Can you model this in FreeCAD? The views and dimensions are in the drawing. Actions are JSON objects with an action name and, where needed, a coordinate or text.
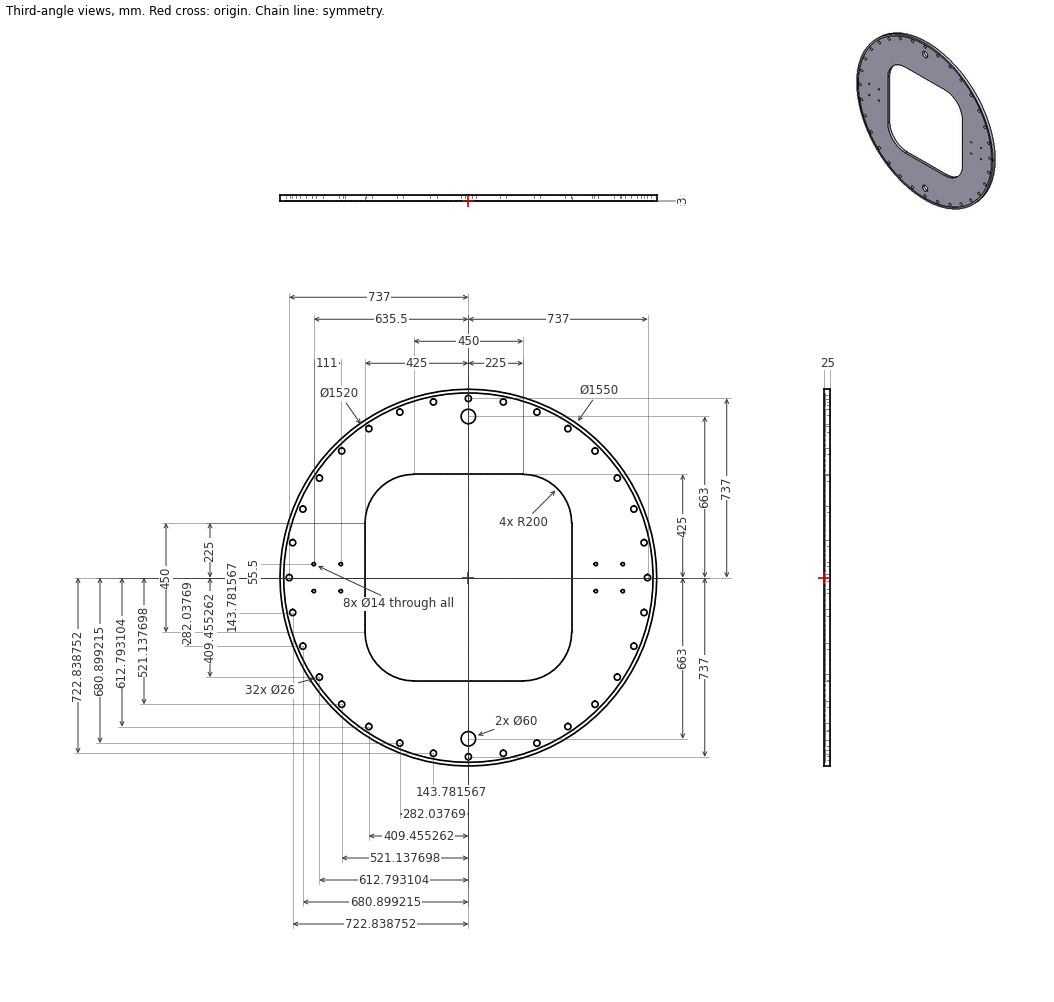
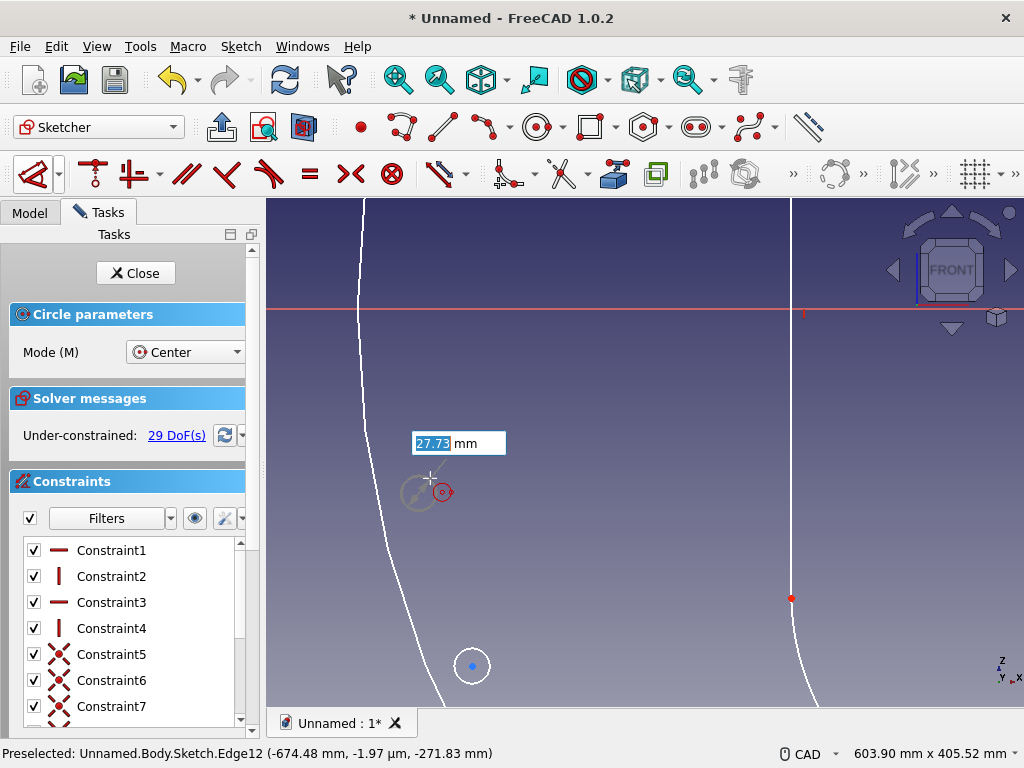
{"action": "left_click", "coordinate": [430, 478]}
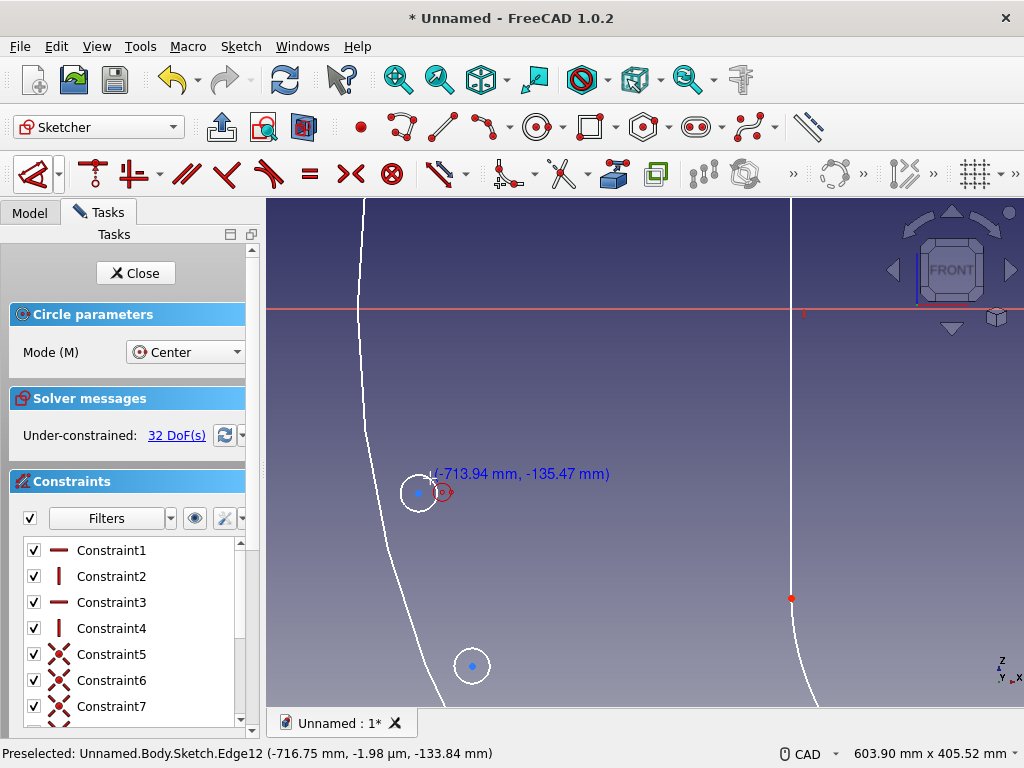
{"action": "scroll", "coordinate": [428, 481], "scroll_direction": "down", "scroll_amount": 9}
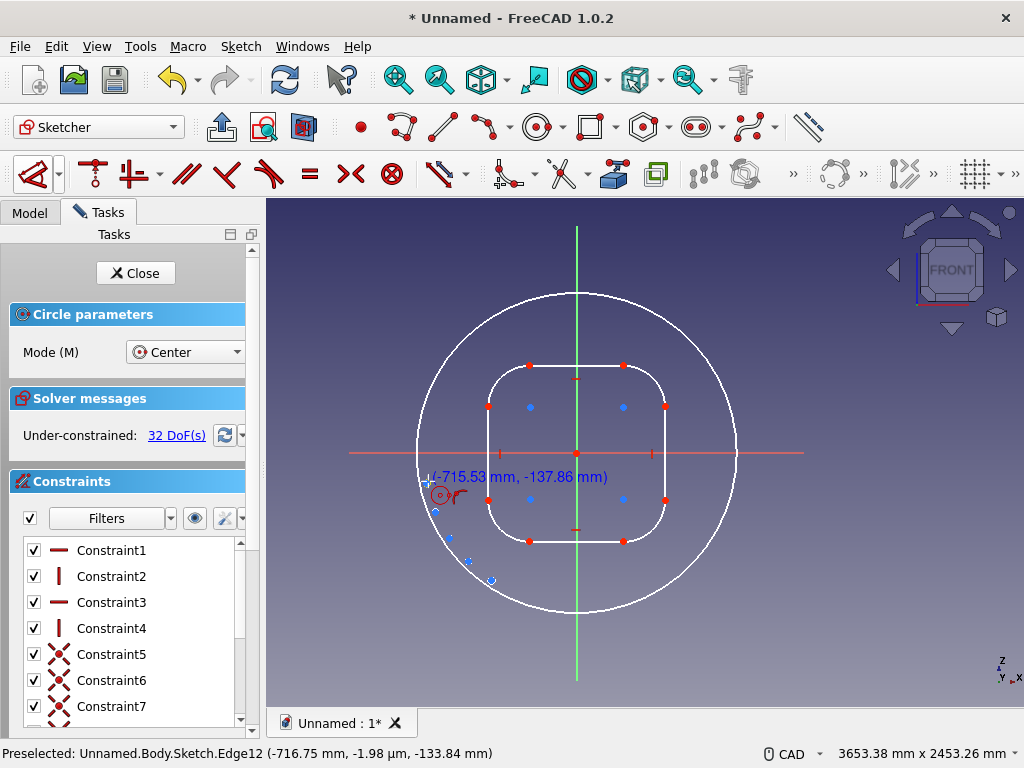
{"action": "scroll", "coordinate": [518, 594], "scroll_direction": "up", "scroll_amount": 11}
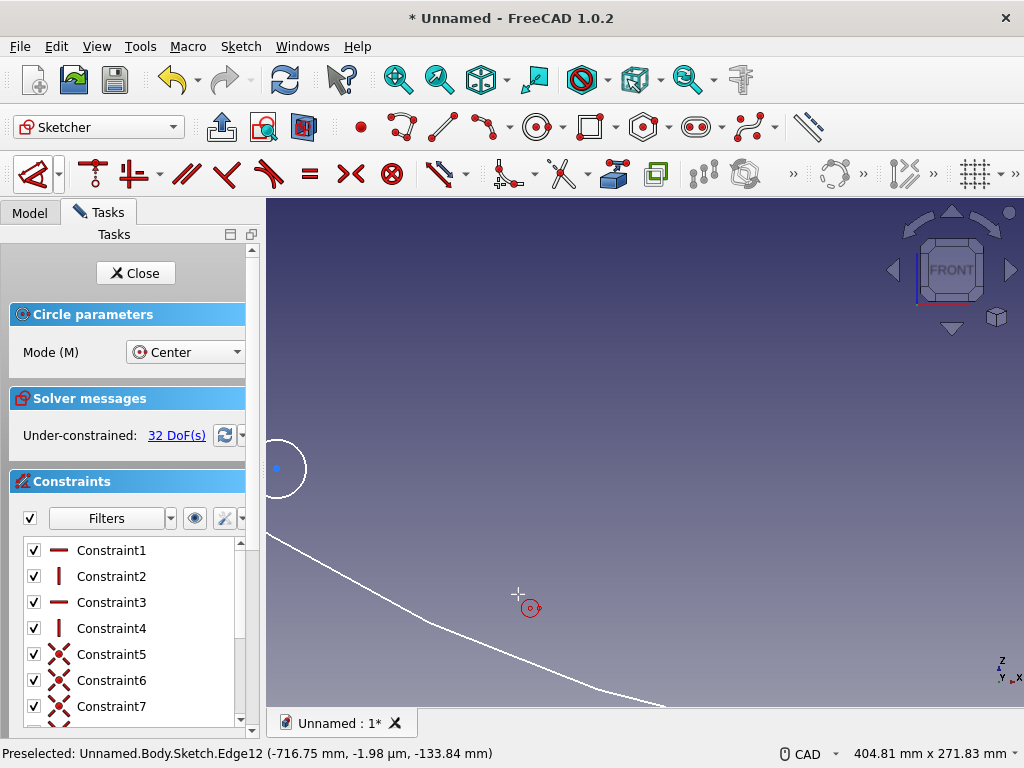
{"action": "scroll", "coordinate": [518, 594], "scroll_direction": "down", "scroll_amount": 11}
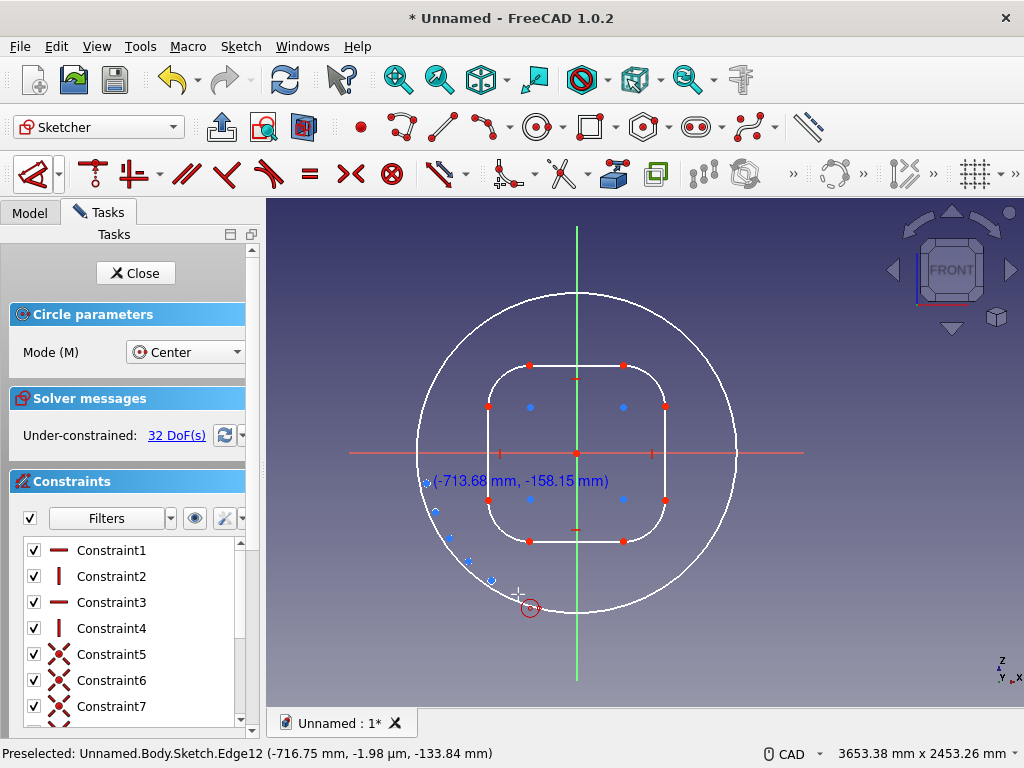
{"action": "scroll", "coordinate": [518, 594], "scroll_direction": "up", "scroll_amount": 4}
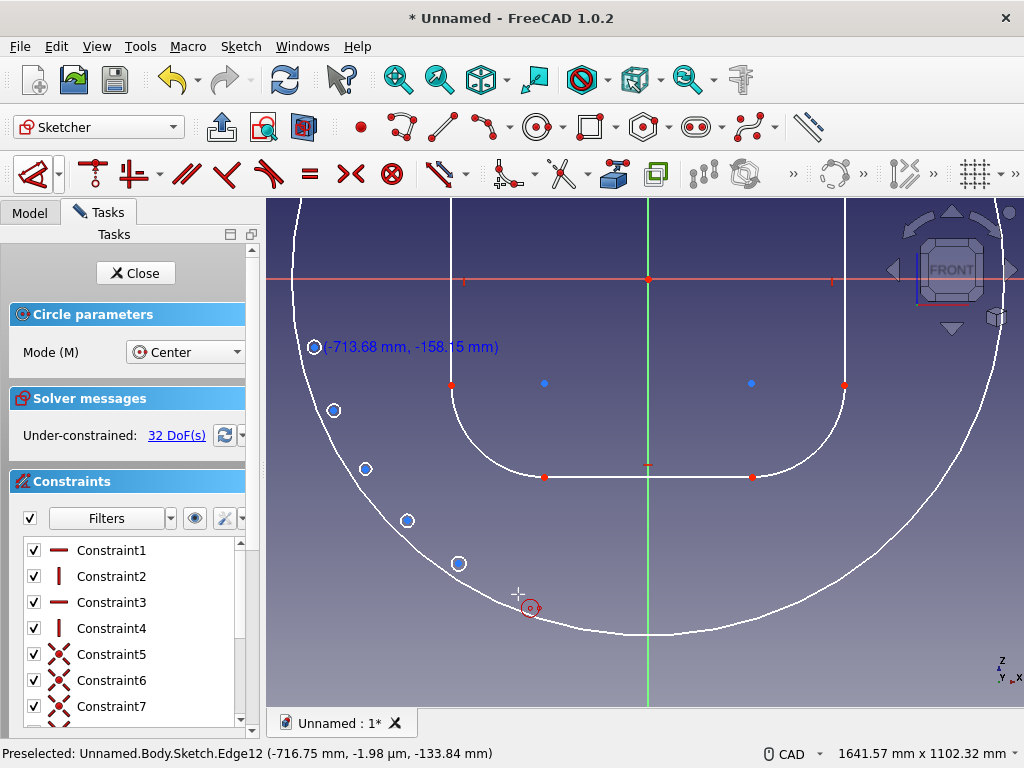
{"action": "left_click", "coordinate": [518, 594]}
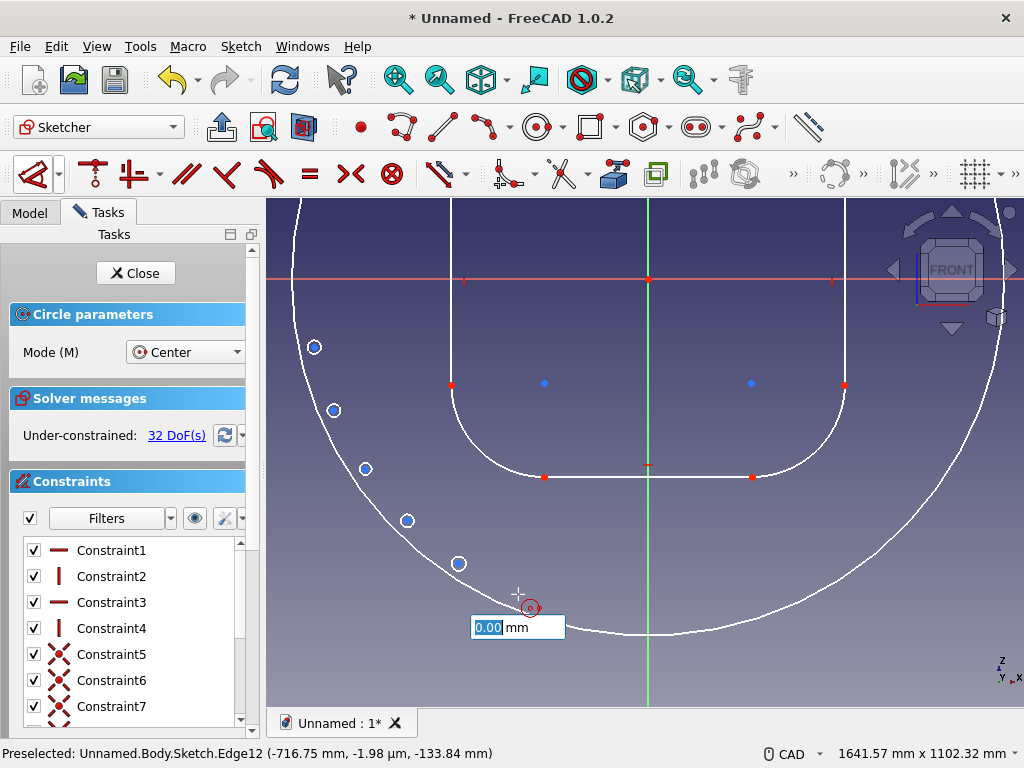
{"action": "scroll", "coordinate": [522, 589], "scroll_direction": "up", "scroll_amount": 5}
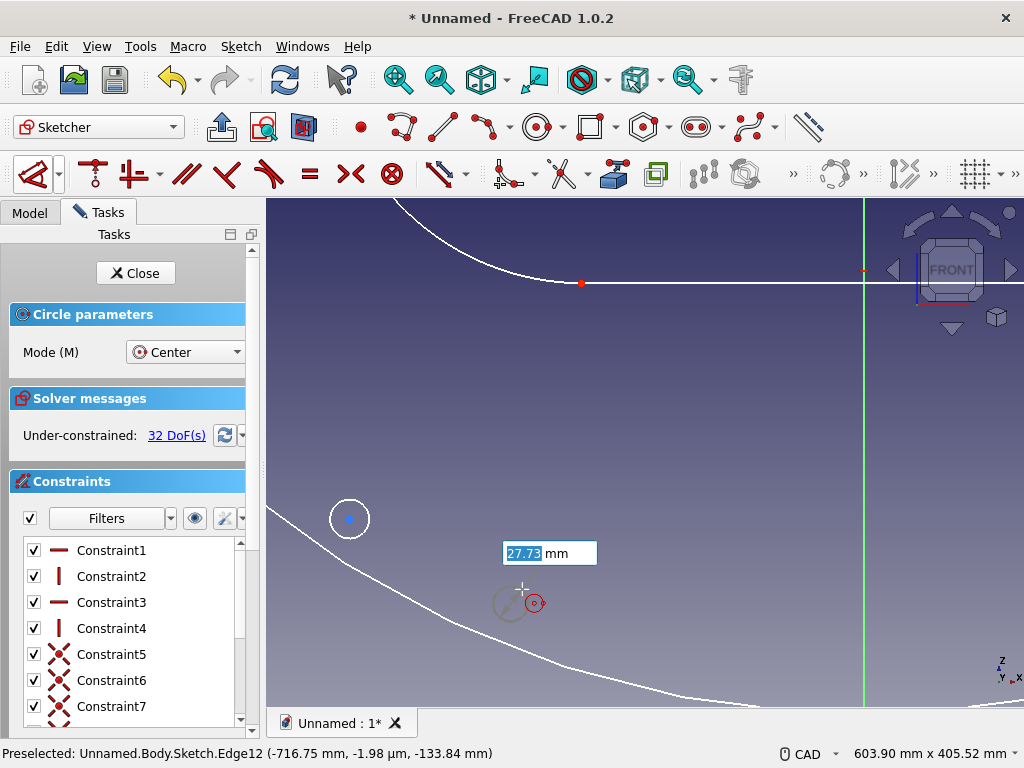
{"action": "left_click", "coordinate": [522, 589]}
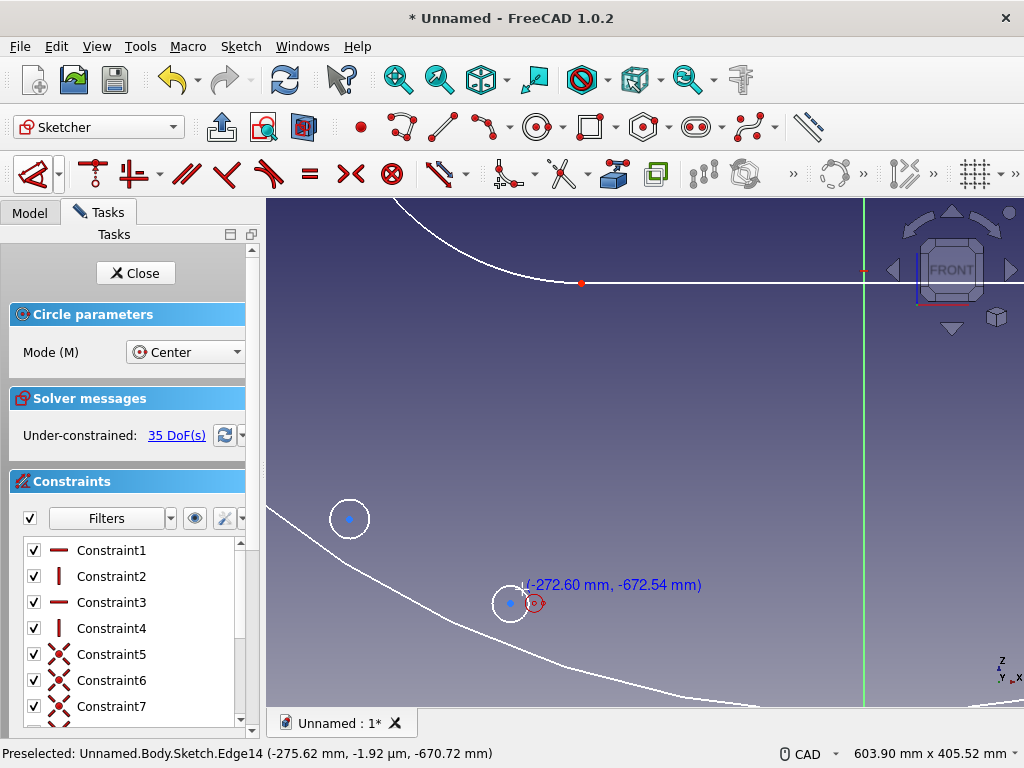
{"action": "scroll", "coordinate": [684, 653], "scroll_direction": "up", "scroll_amount": 2}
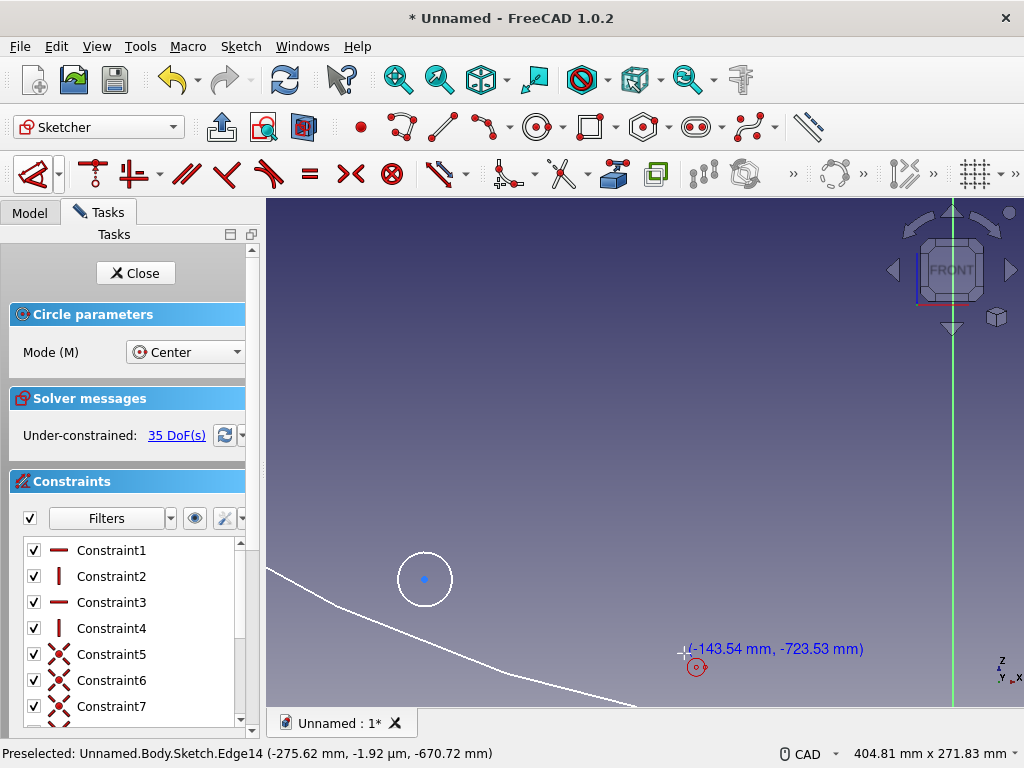
{"action": "scroll", "coordinate": [530, 596], "scroll_direction": "down", "scroll_amount": 11}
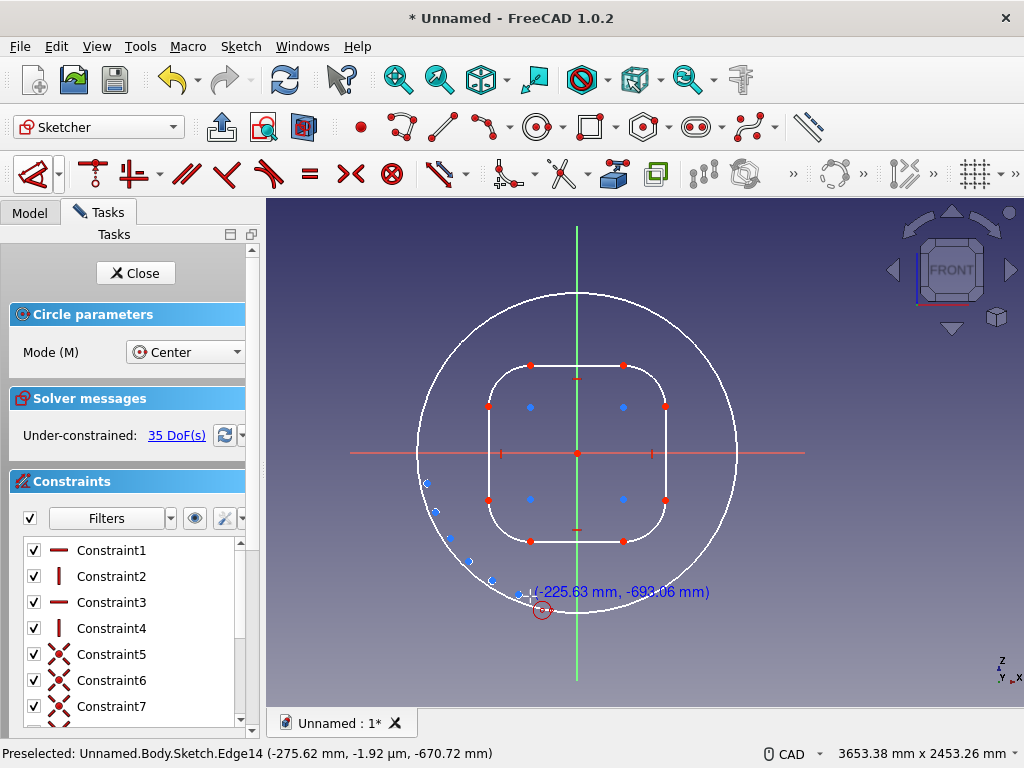
{"action": "scroll", "coordinate": [547, 603], "scroll_direction": "up", "scroll_amount": 4}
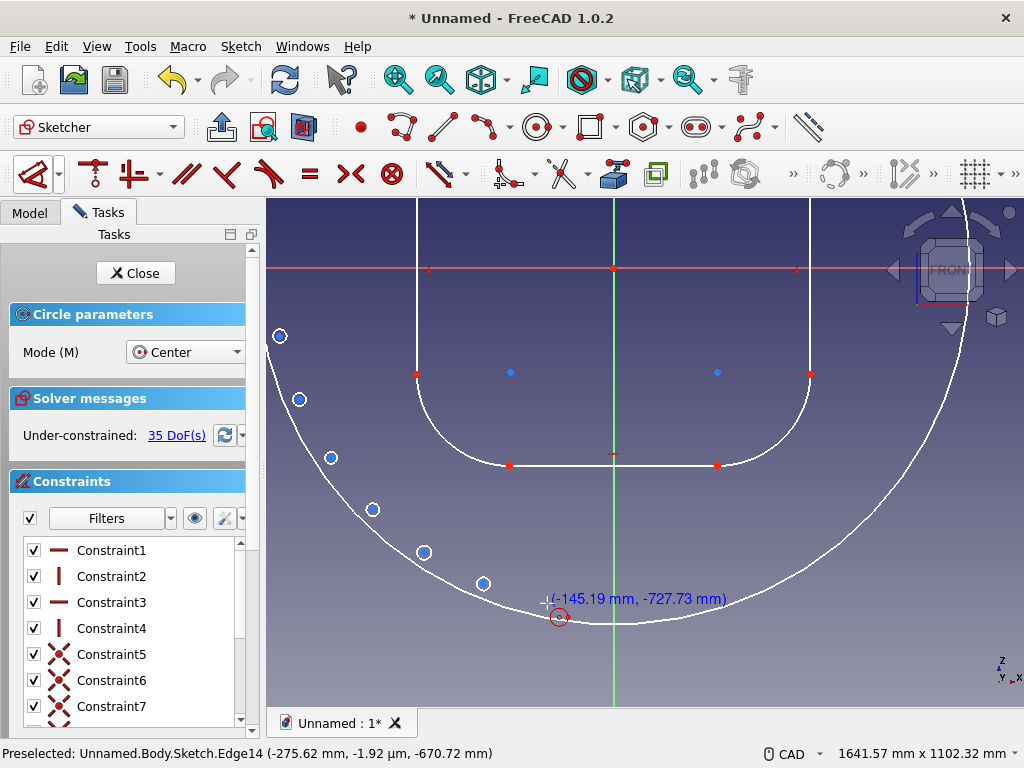
{"action": "left_click", "coordinate": [547, 602]}